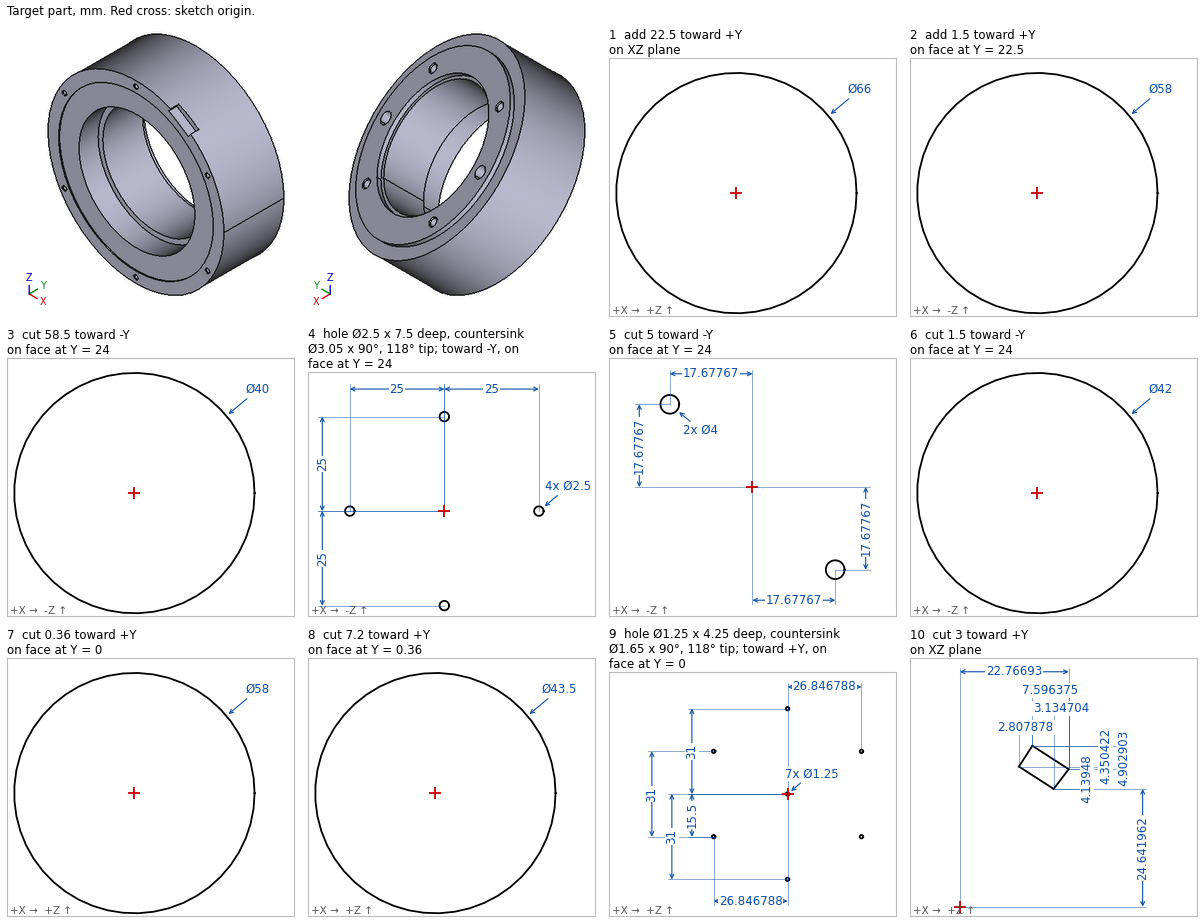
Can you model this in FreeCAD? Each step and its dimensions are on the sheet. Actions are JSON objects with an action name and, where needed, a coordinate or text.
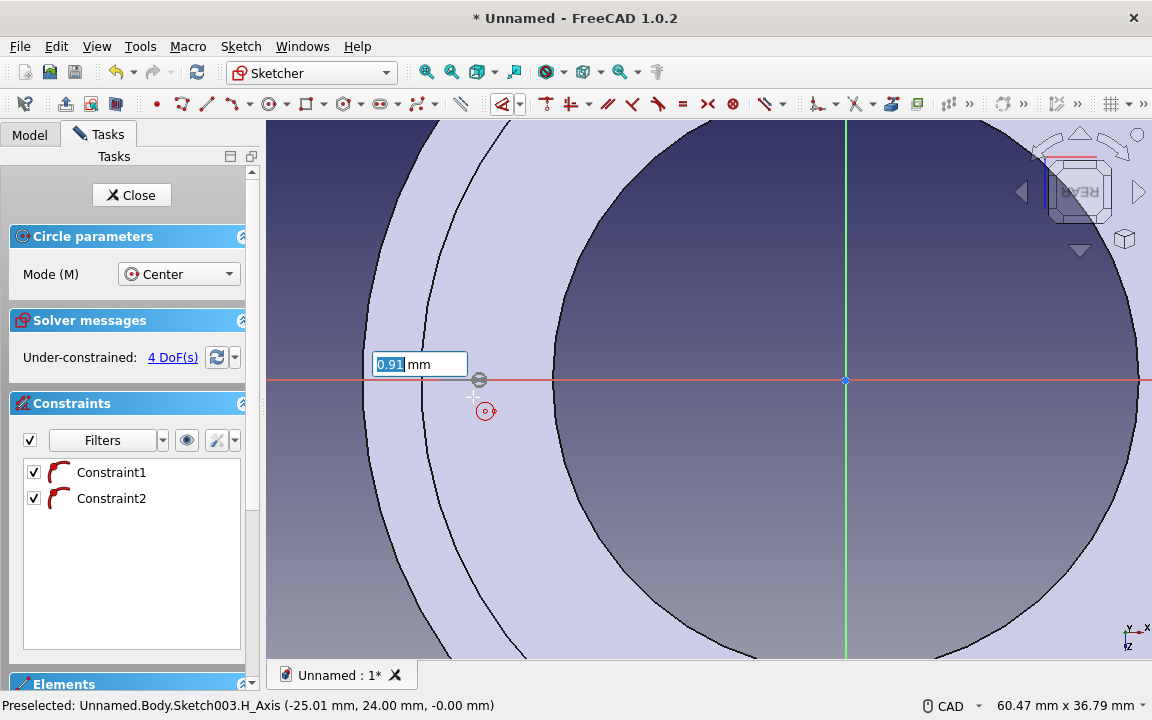
{"action": "left_click", "coordinate": [473, 397]}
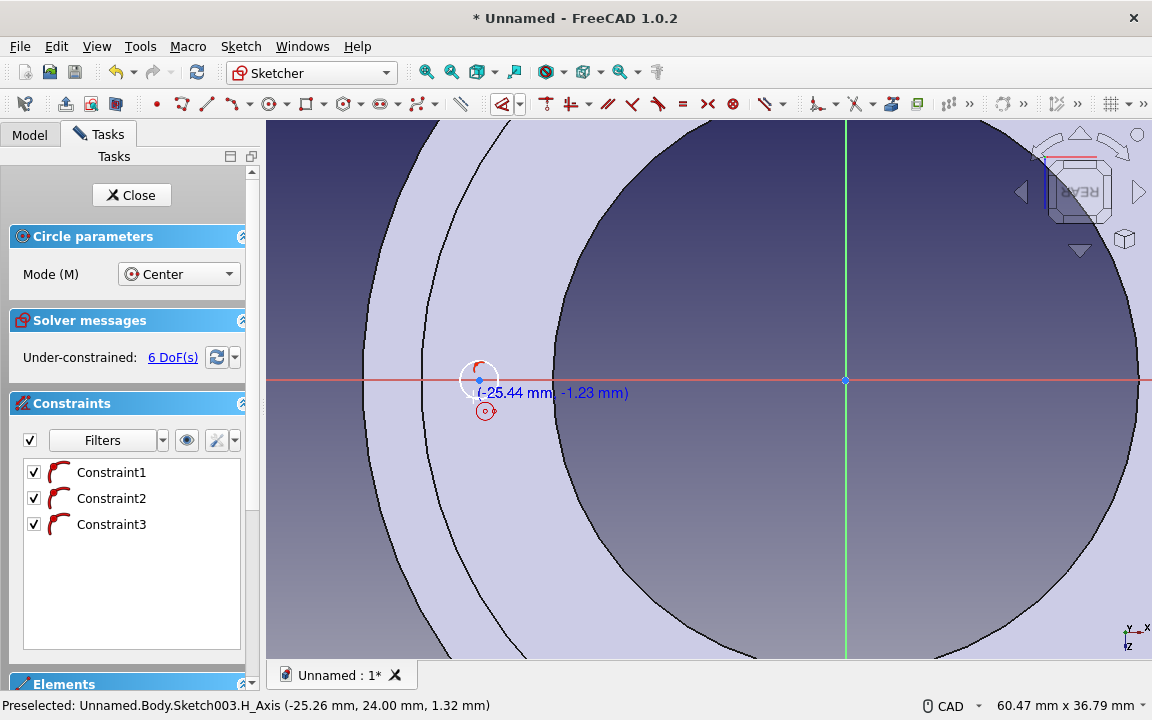
{"action": "scroll", "coordinate": [473, 397], "scroll_direction": "down", "scroll_amount": 4}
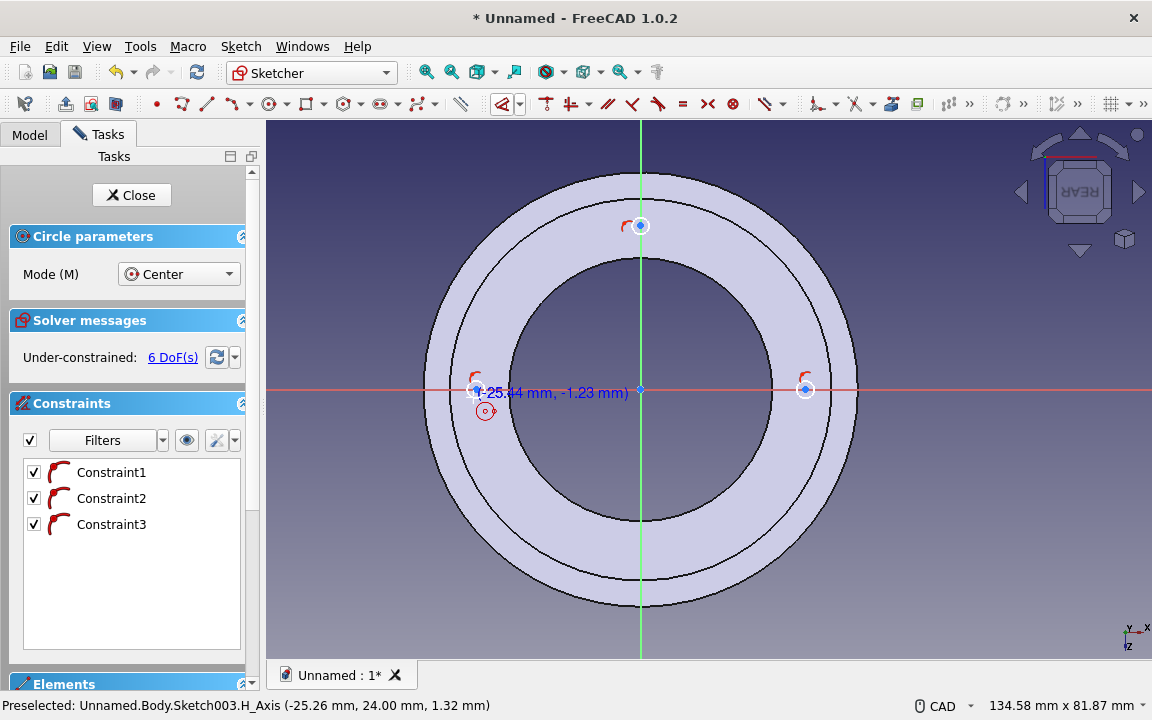
{"action": "scroll", "coordinate": [641, 554], "scroll_direction": "up", "scroll_amount": 6}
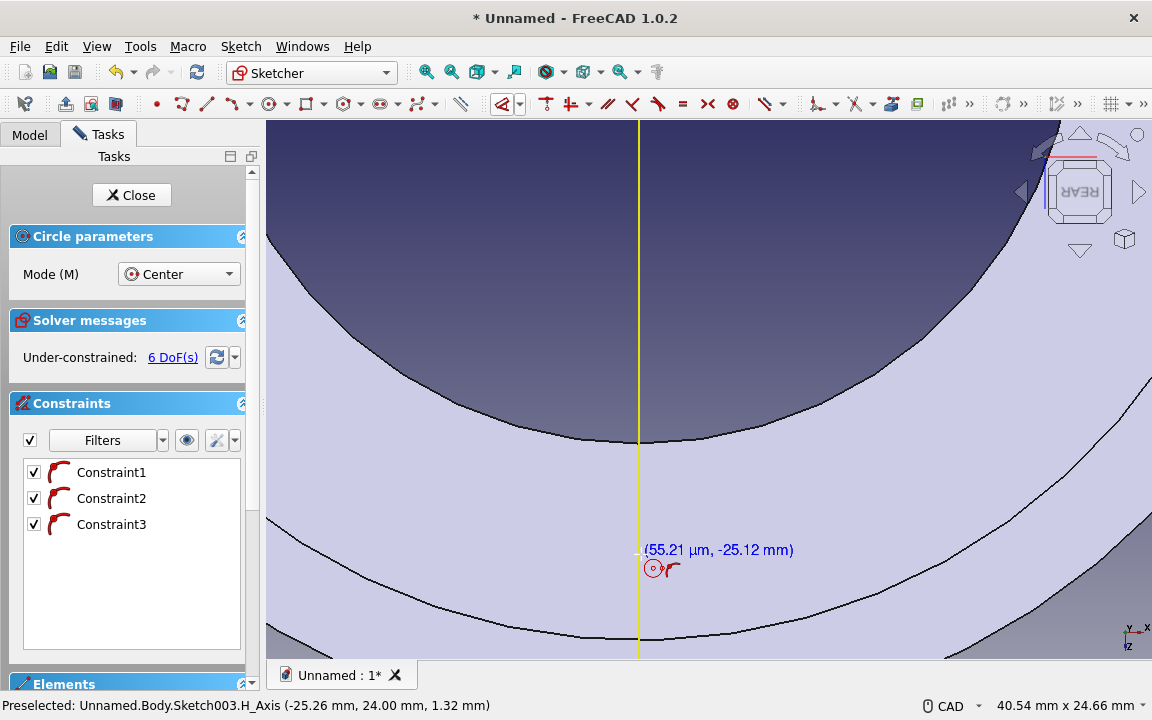
{"action": "scroll", "coordinate": [641, 555], "scroll_direction": "down", "scroll_amount": 6}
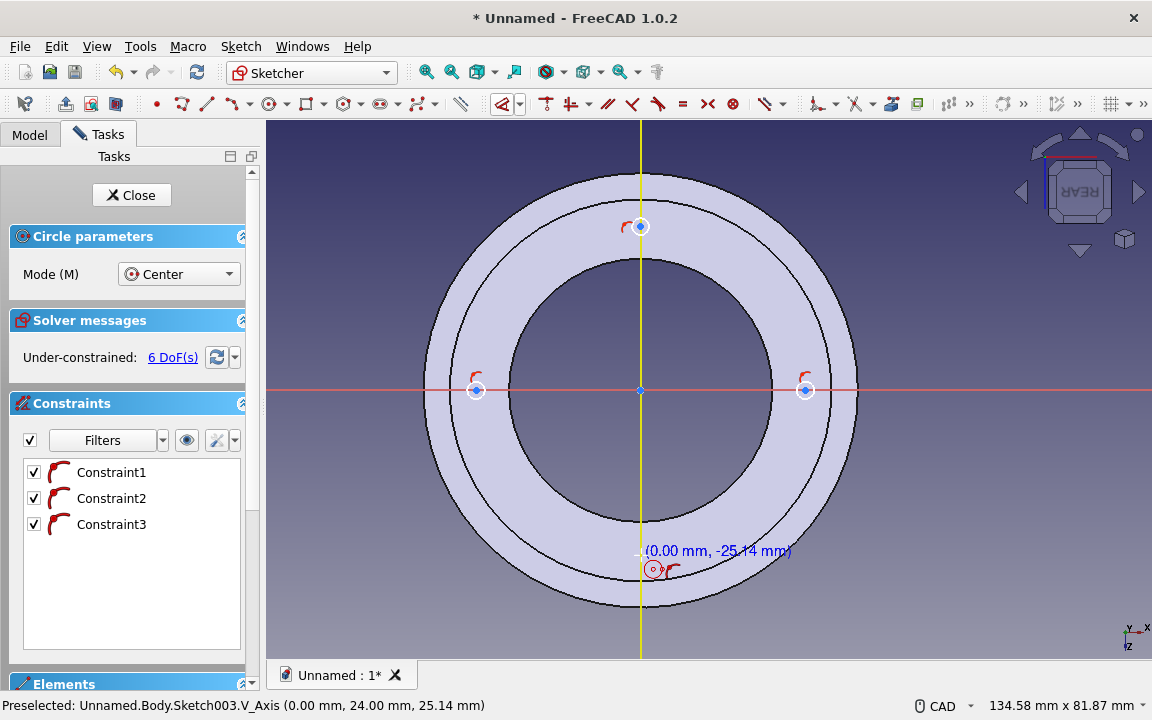
{"action": "left_click", "coordinate": [641, 555]}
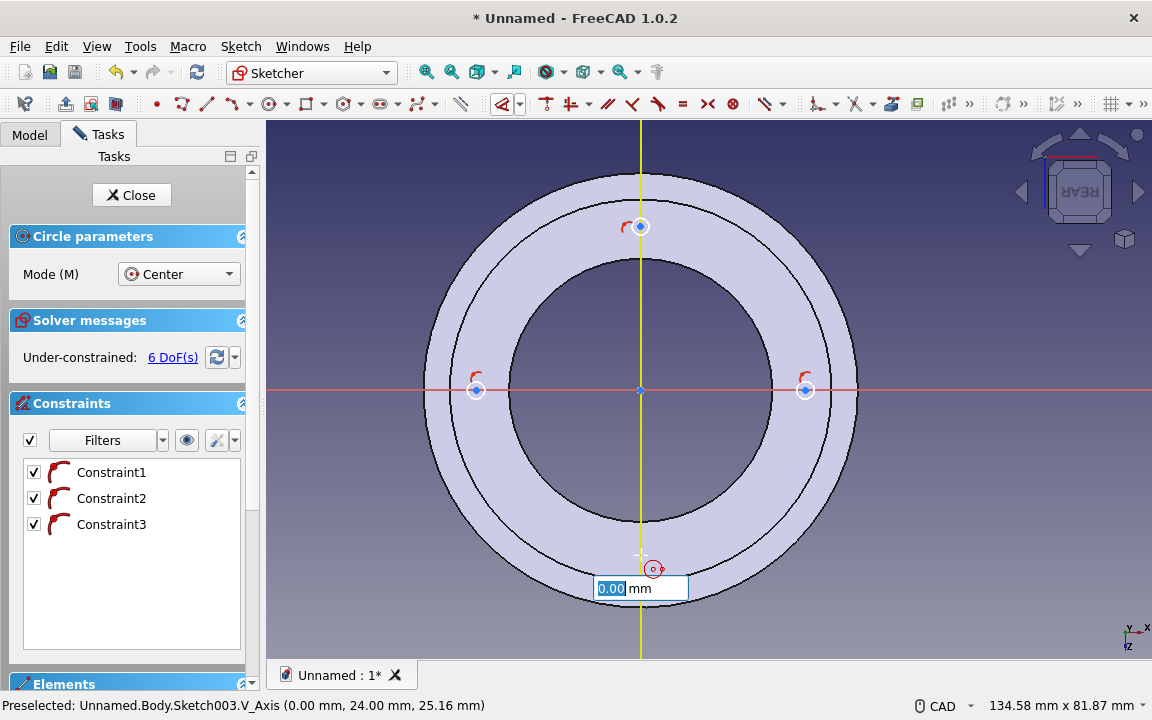
{"action": "scroll", "coordinate": [648, 552], "scroll_direction": "up", "scroll_amount": 4}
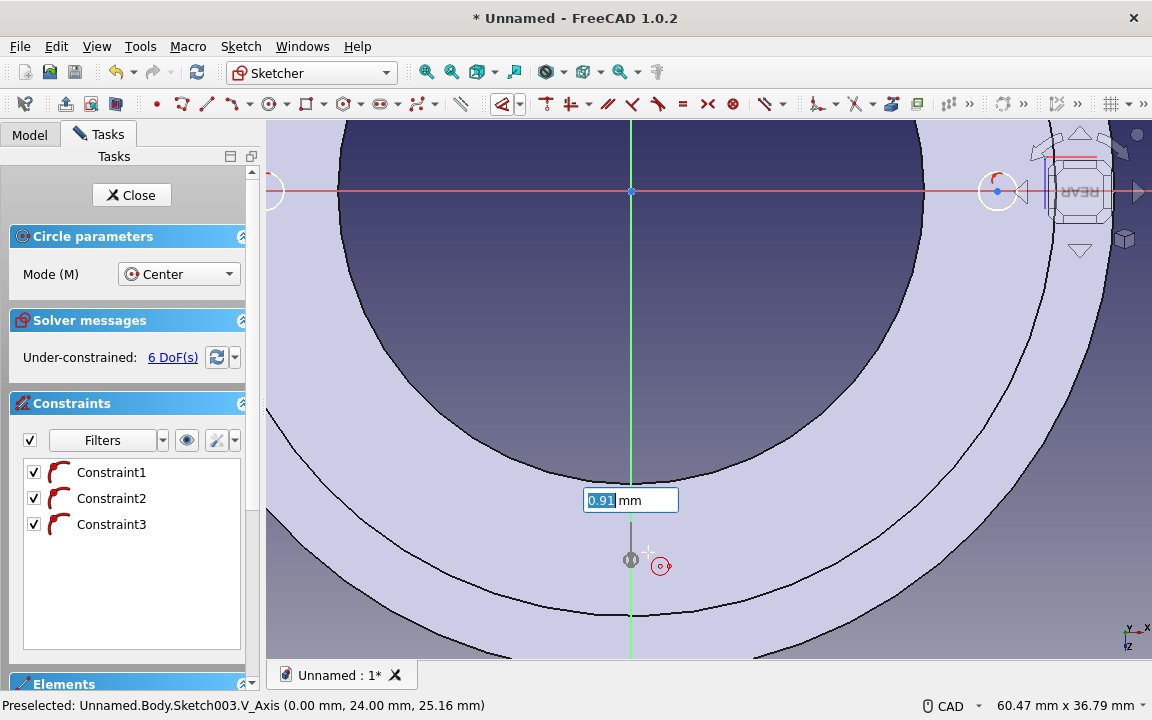
{"action": "left_click", "coordinate": [648, 551]}
{"action": "key", "text": "Escape"}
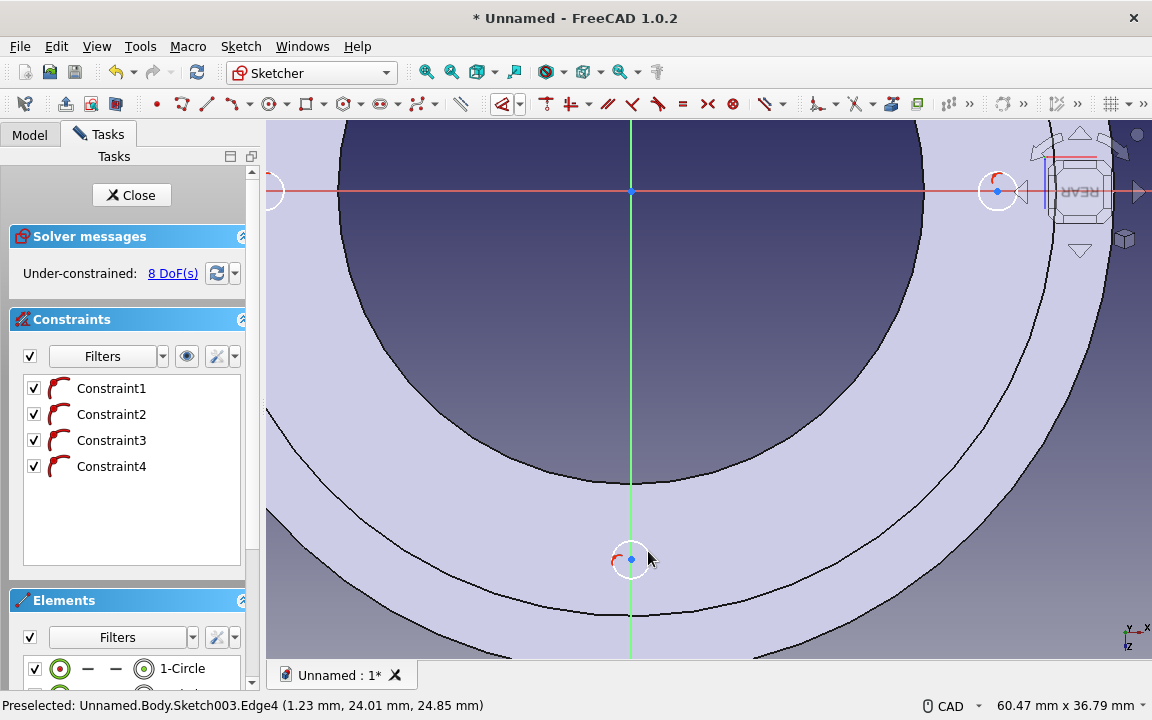
{"action": "left_click", "coordinate": [984, 178]}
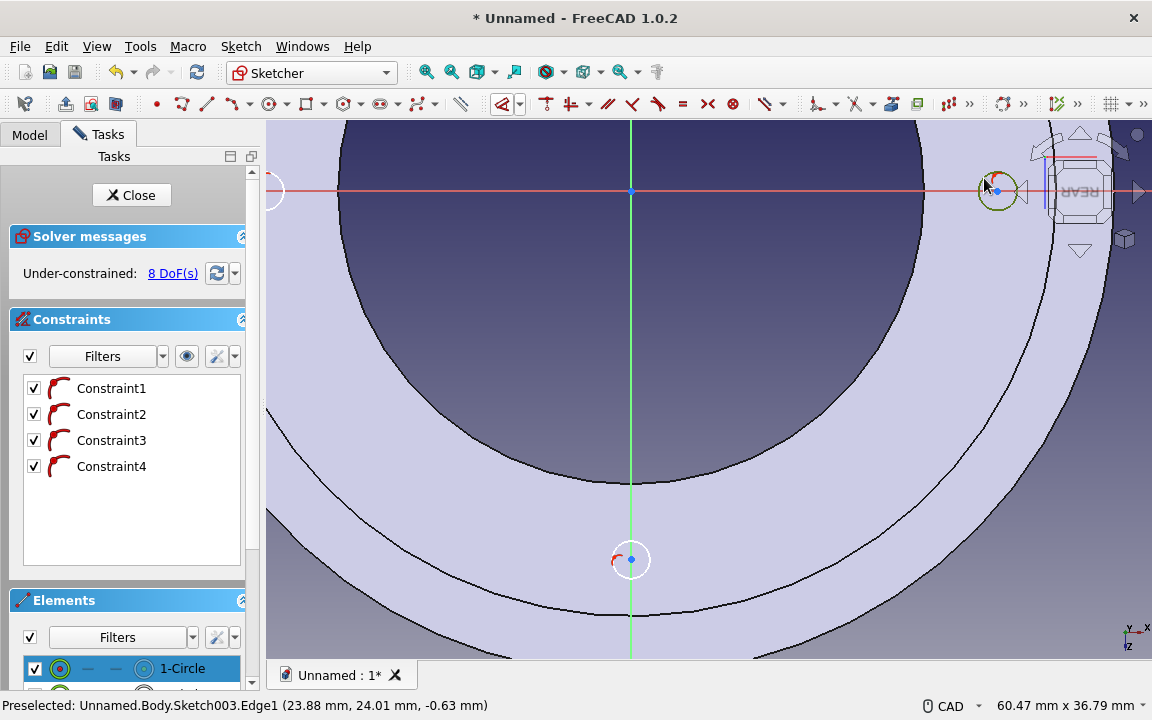
{"action": "scroll", "coordinate": [648, 551], "scroll_direction": "down", "scroll_amount": 4}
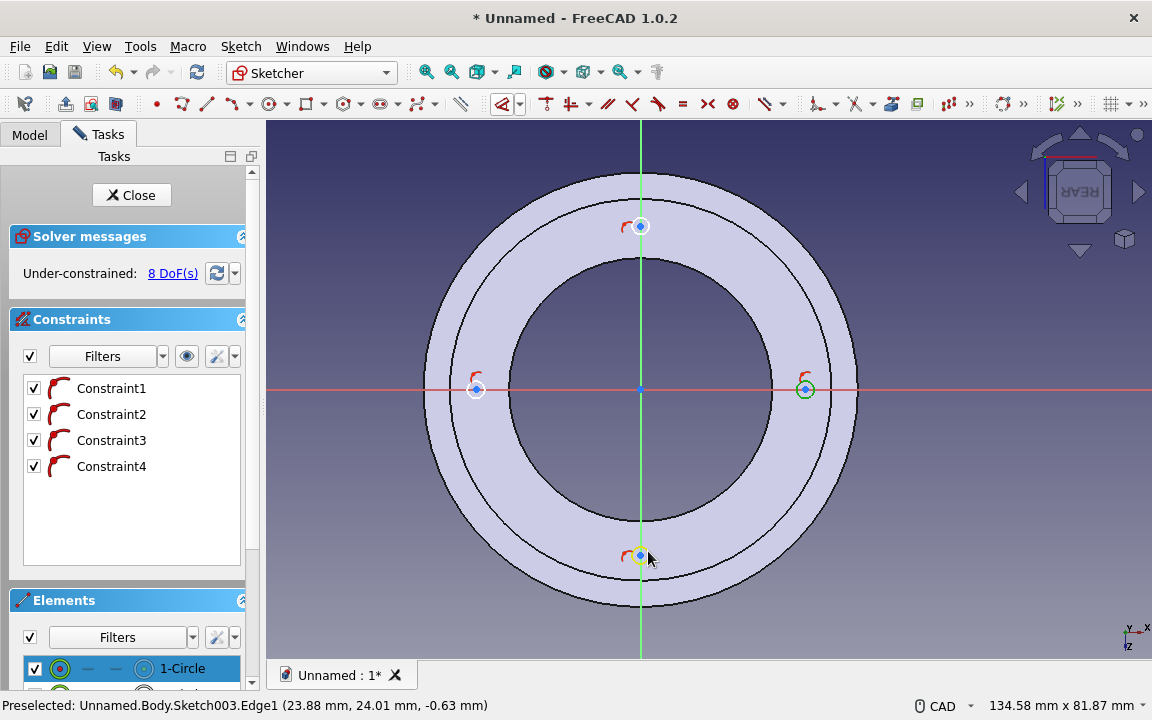
{"action": "scroll", "coordinate": [647, 220], "scroll_direction": "up", "scroll_amount": 5}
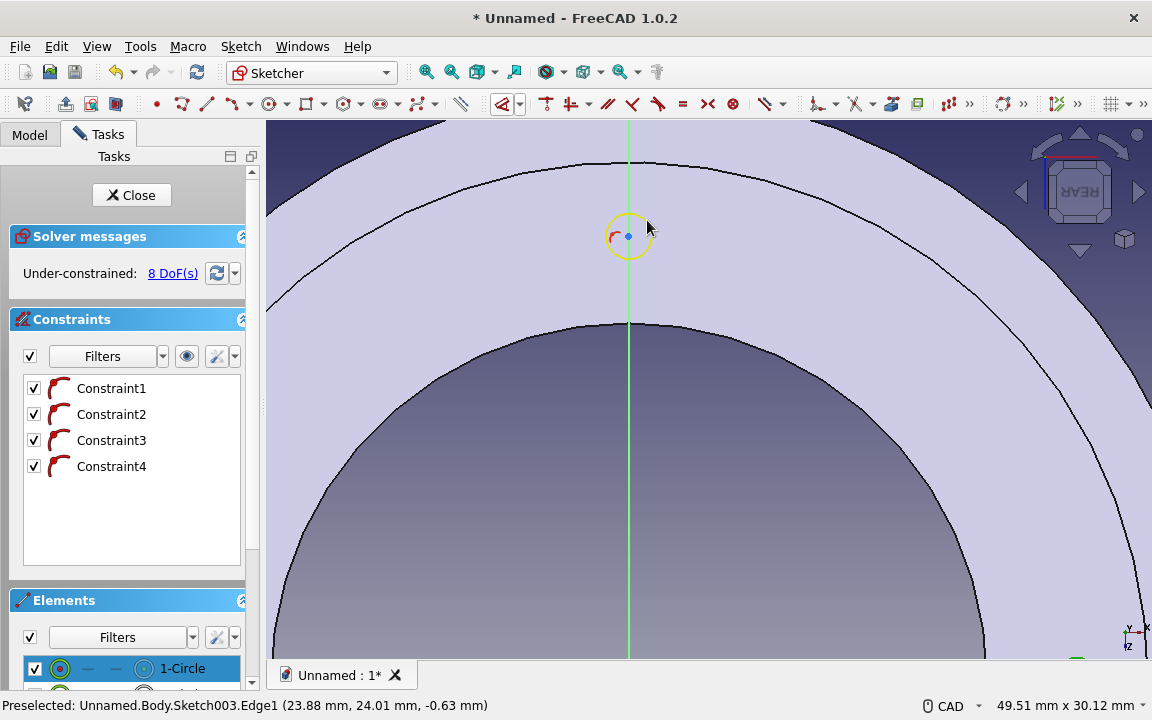
{"action": "left_click", "coordinate": [645, 220]}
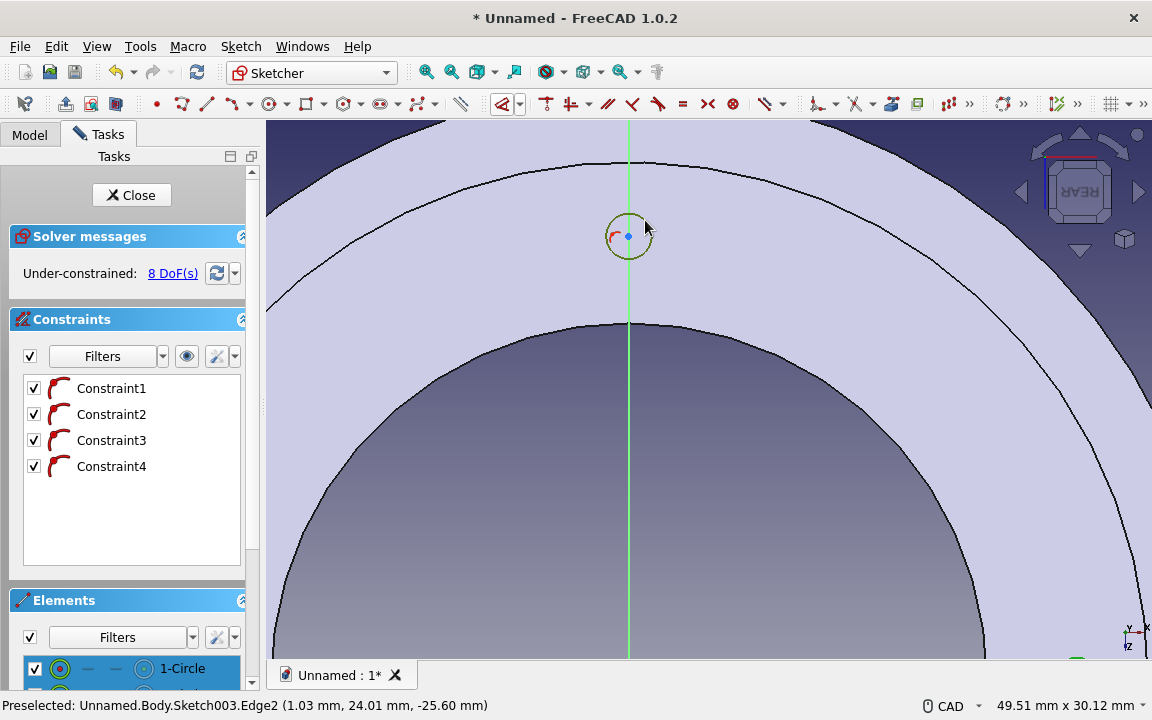
{"action": "scroll", "coordinate": [647, 220], "scroll_direction": "down", "scroll_amount": 5}